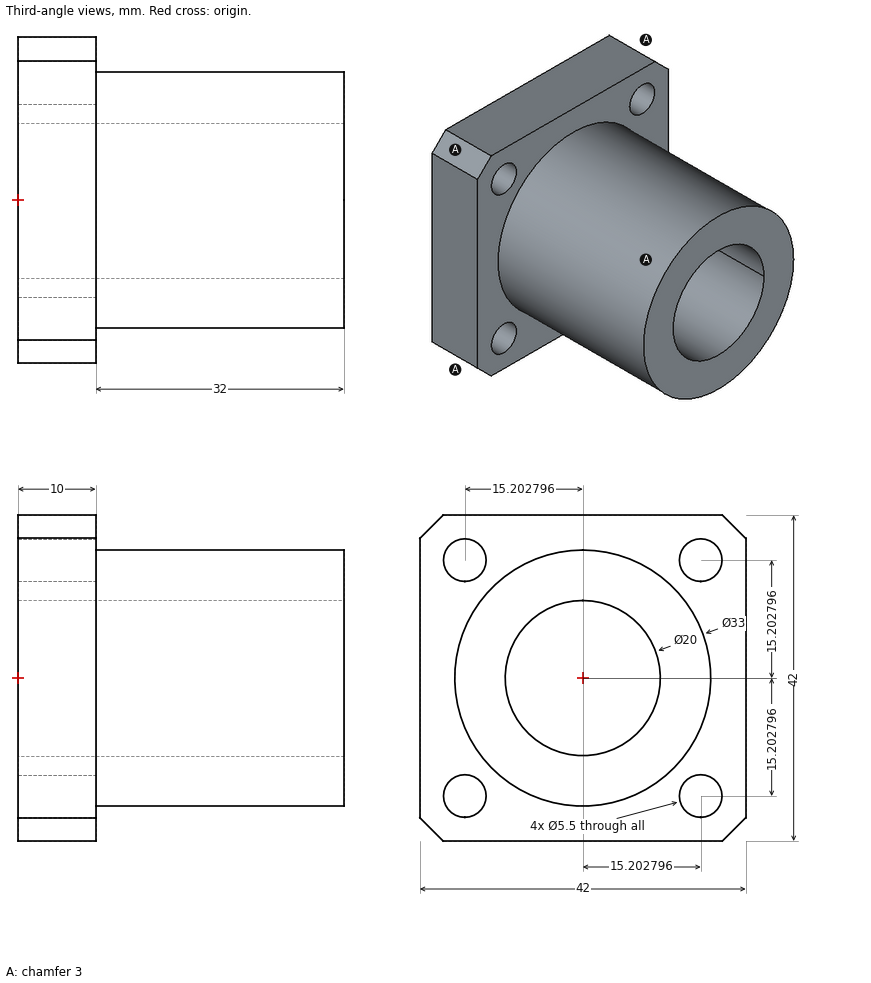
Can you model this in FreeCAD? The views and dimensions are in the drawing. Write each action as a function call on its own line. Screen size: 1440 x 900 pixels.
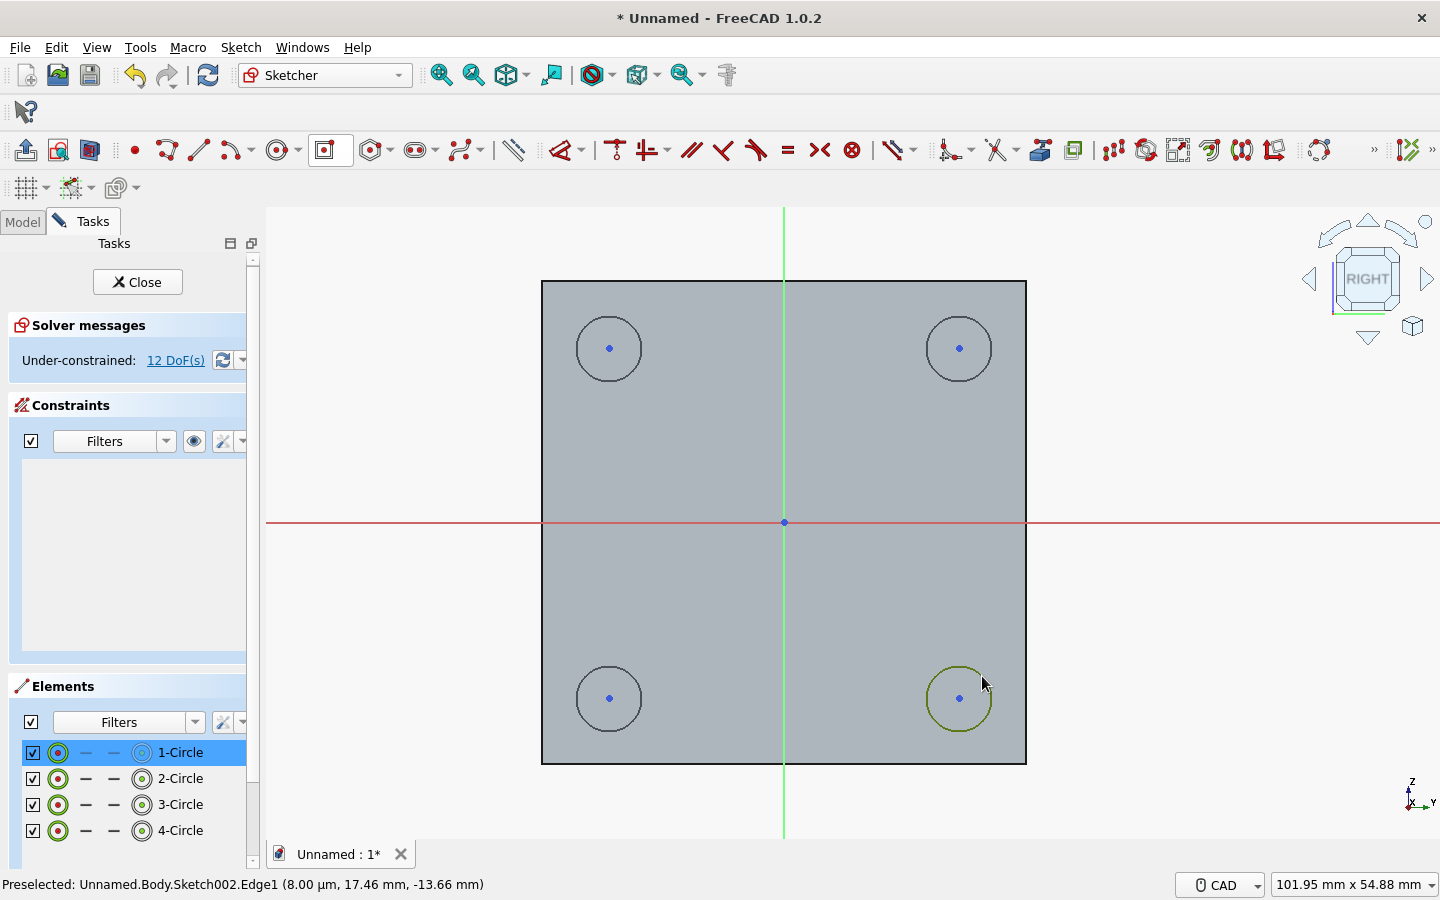
click(982, 326)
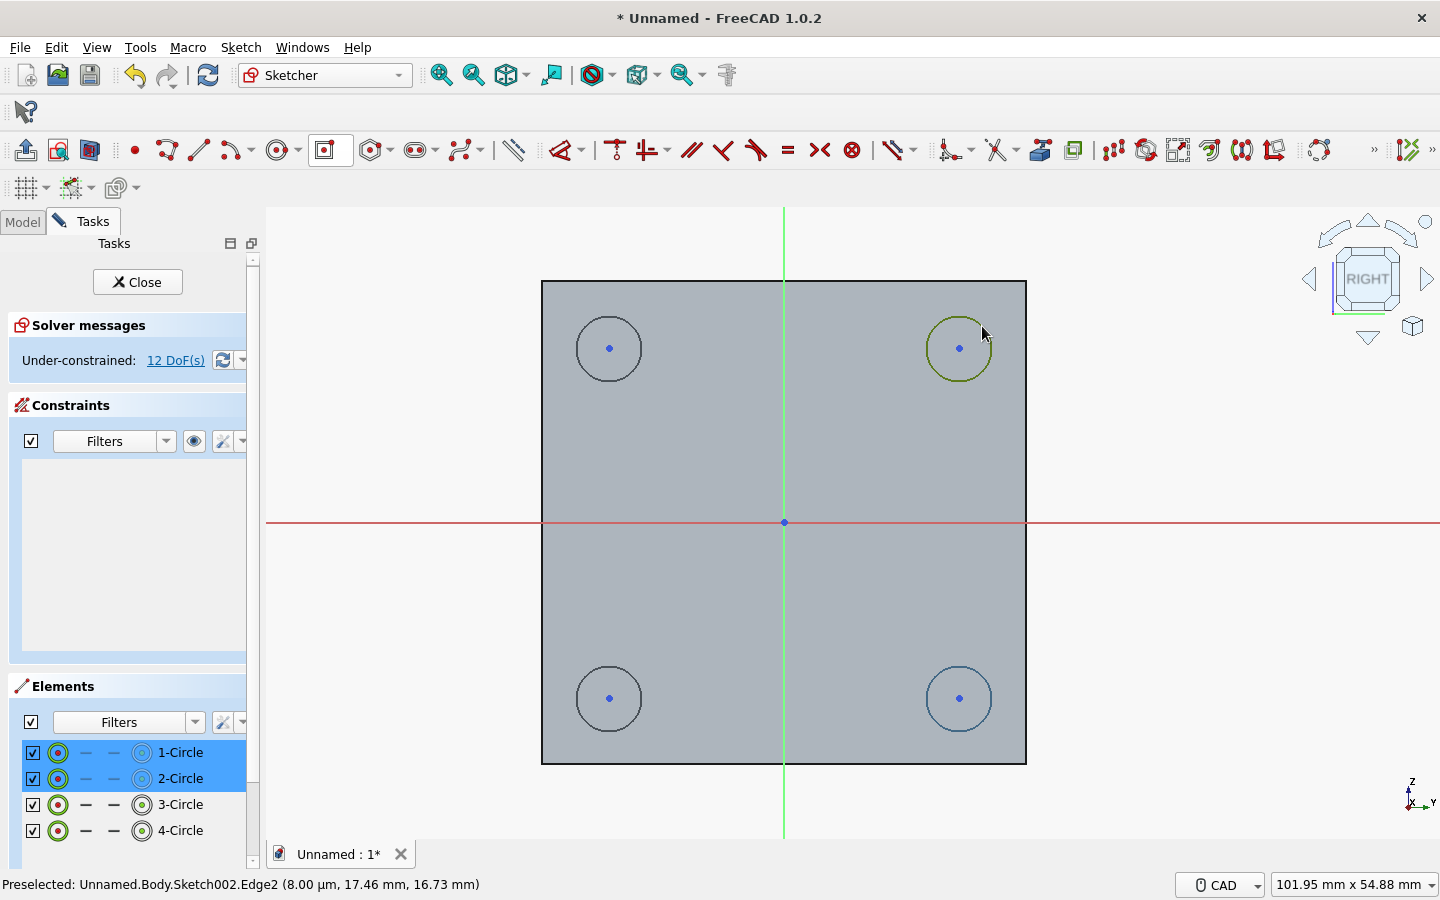
click(632, 326)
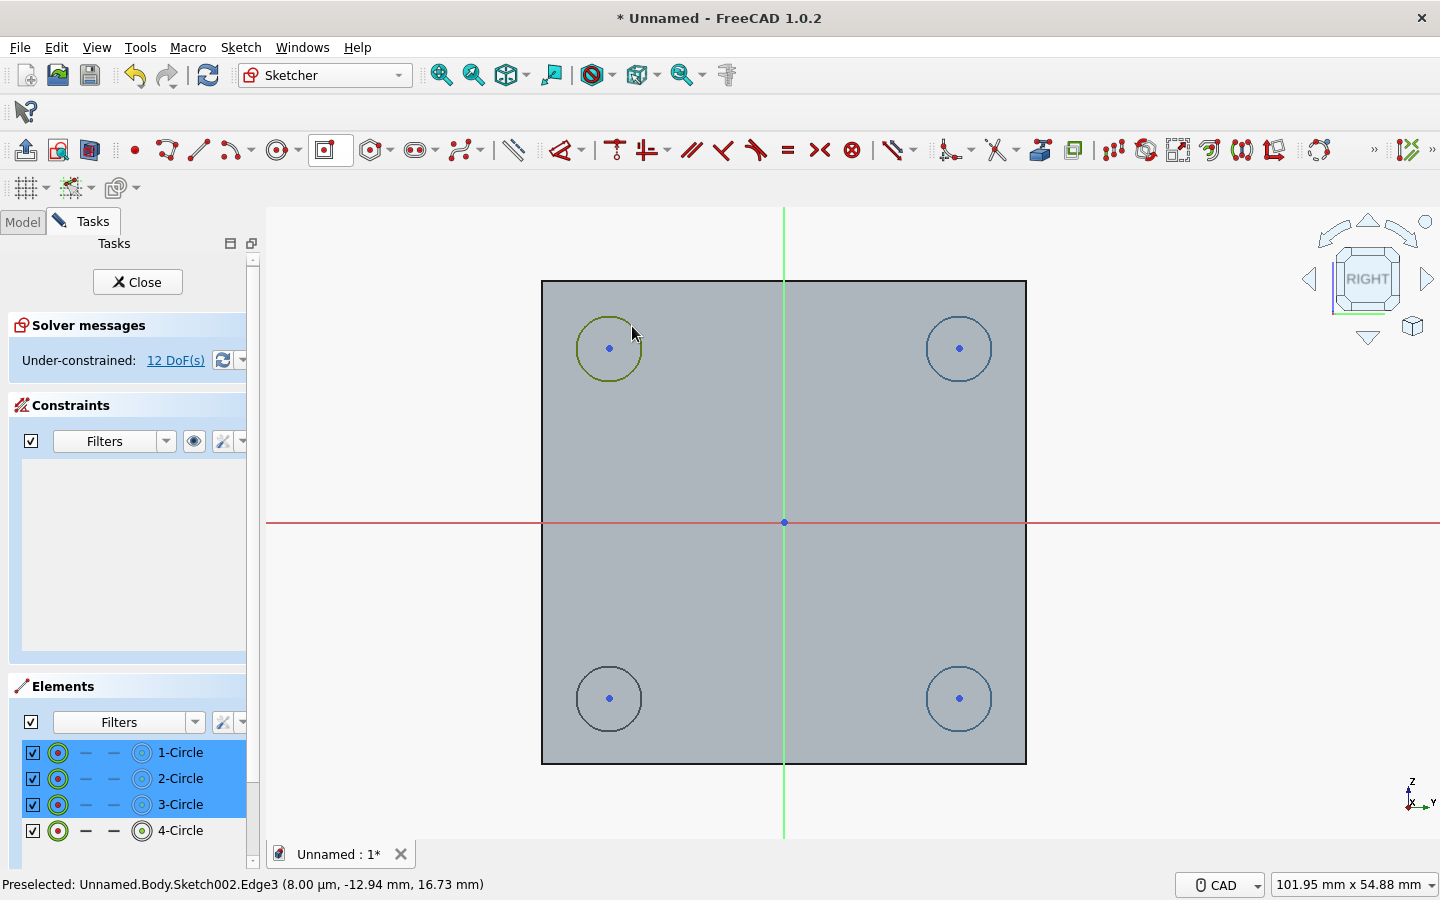
click(632, 676)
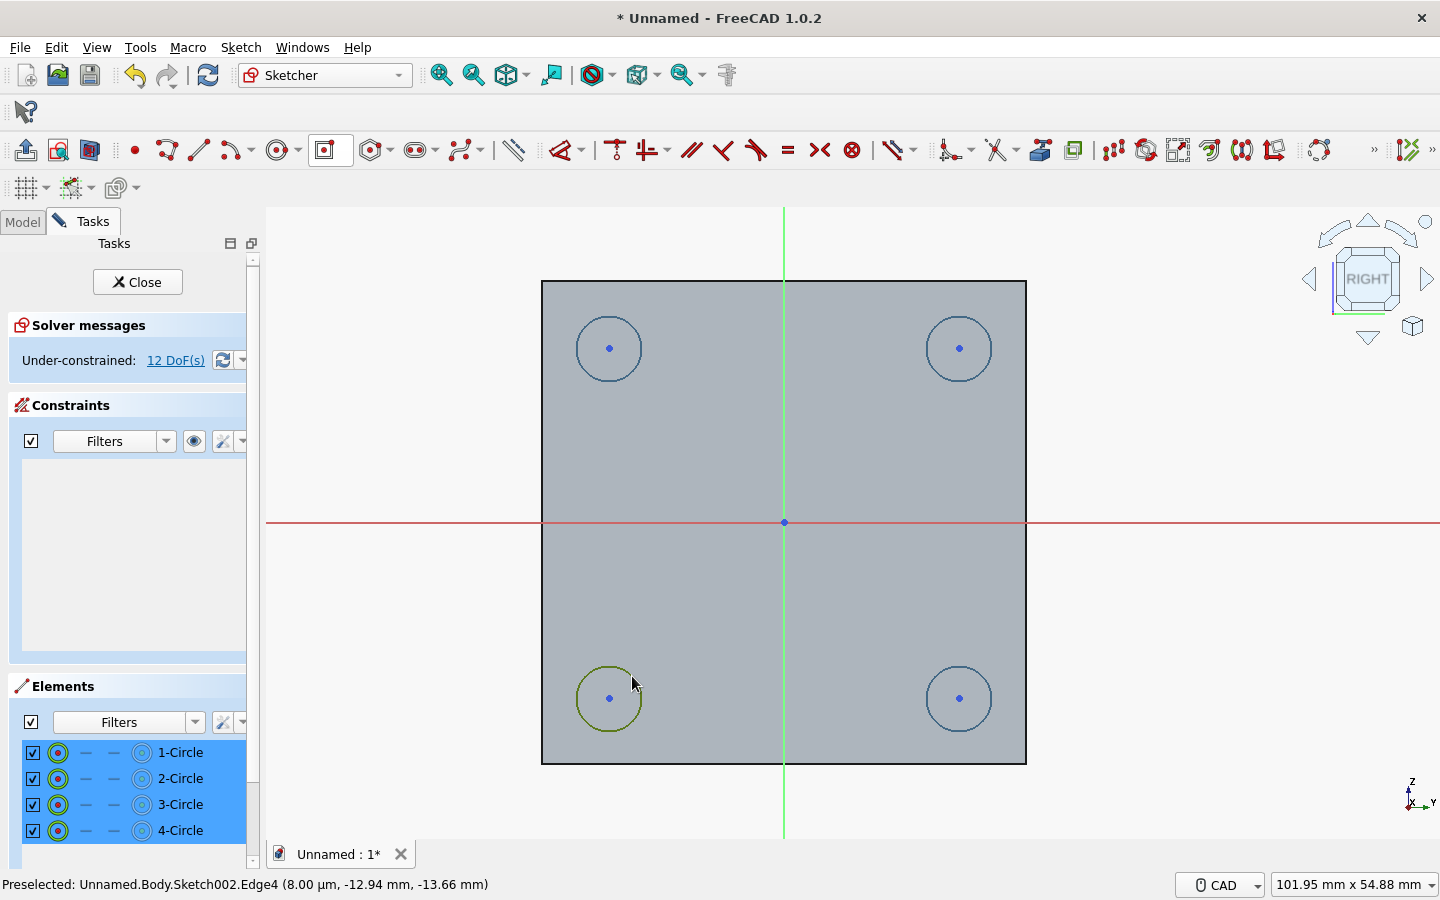
click(788, 150)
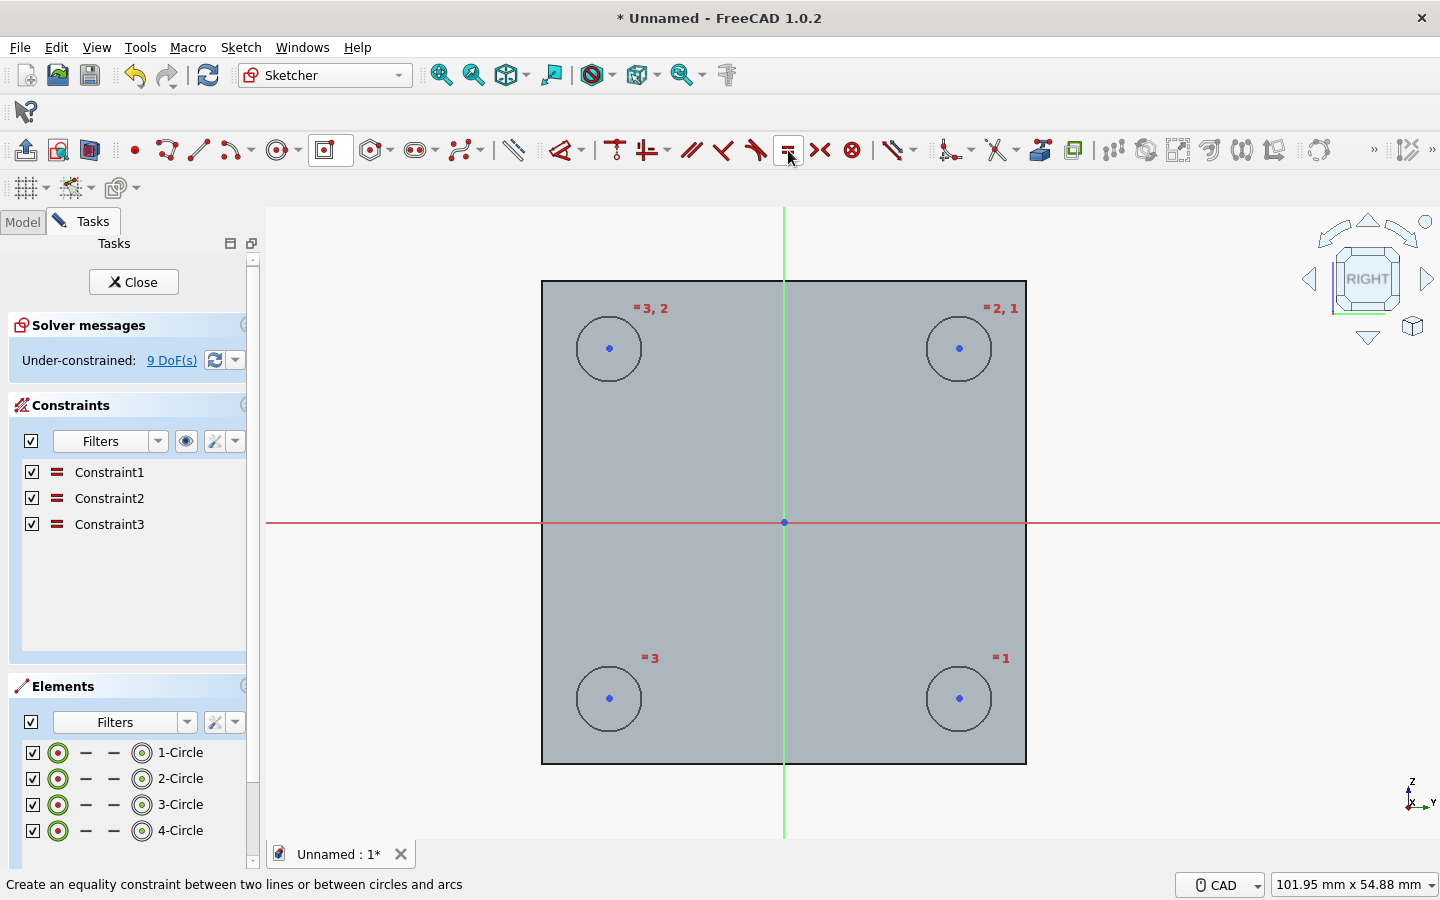
click(560, 150)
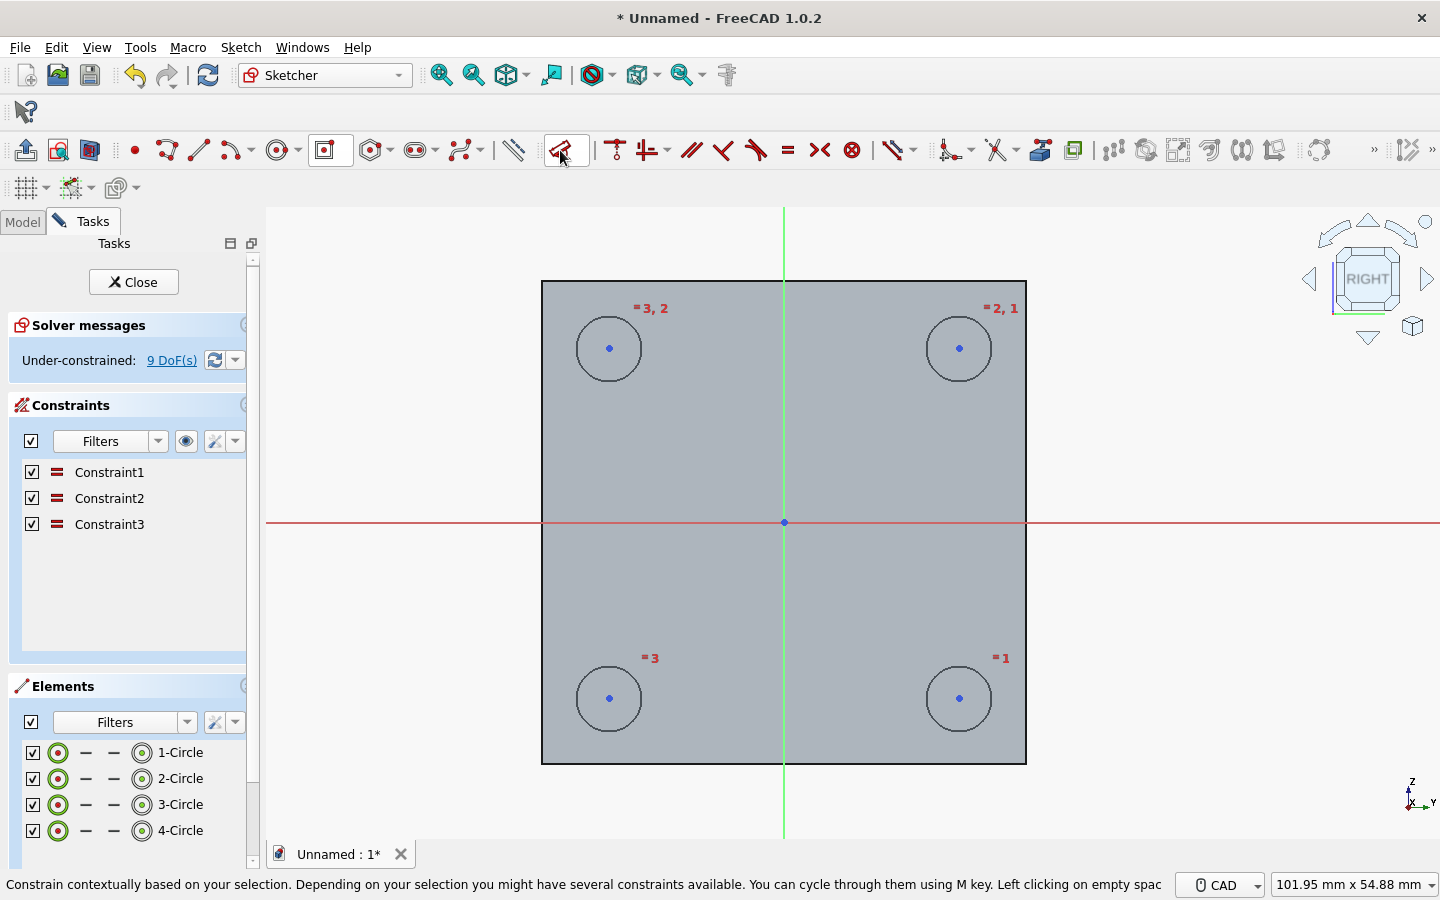
click(982, 676)
click(1005, 653)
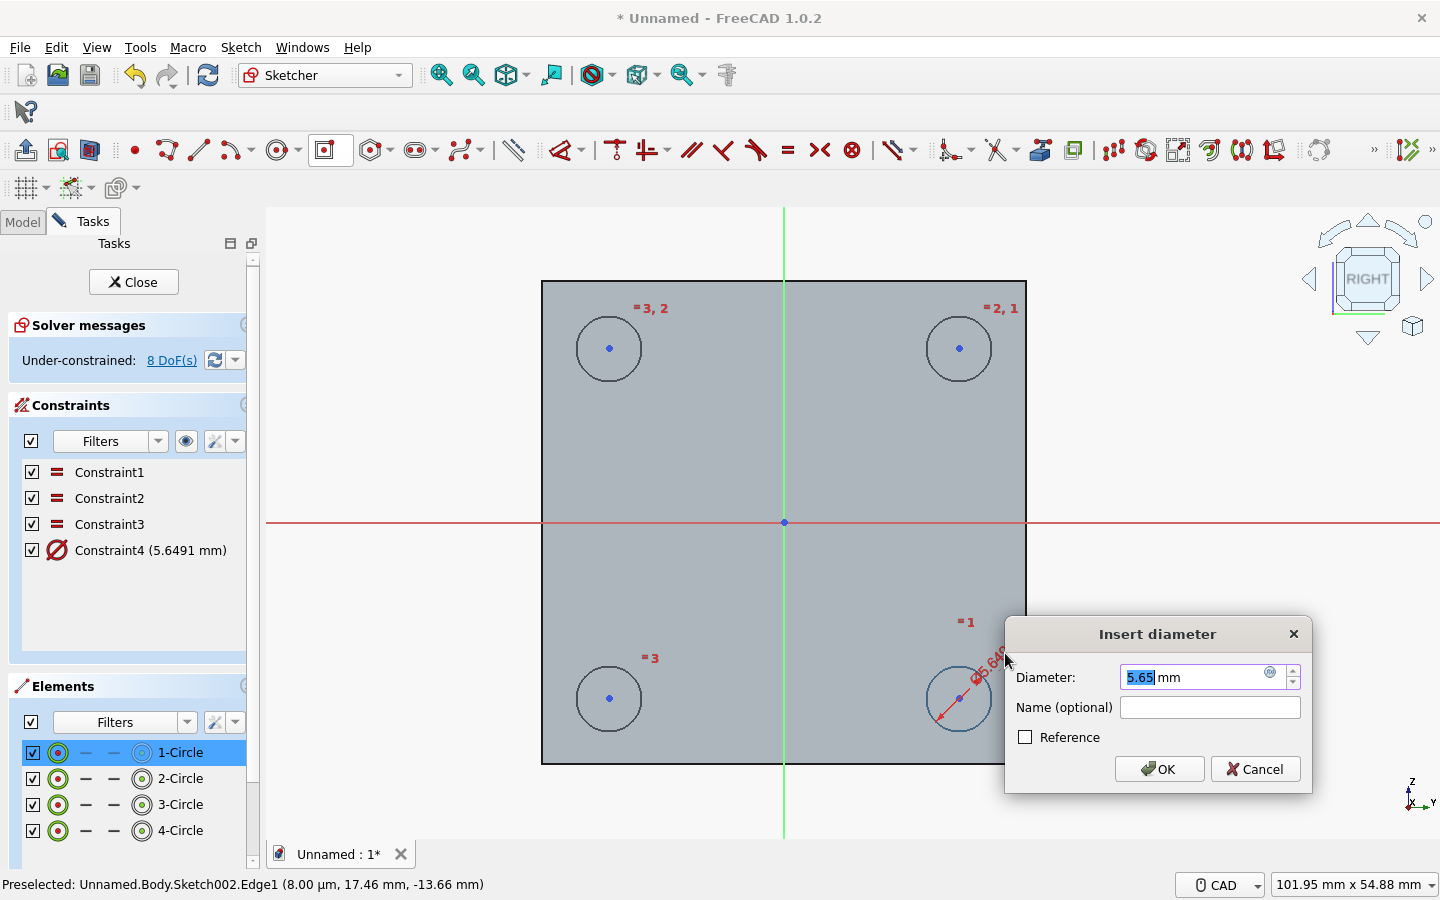
text(5.5)
key(Return)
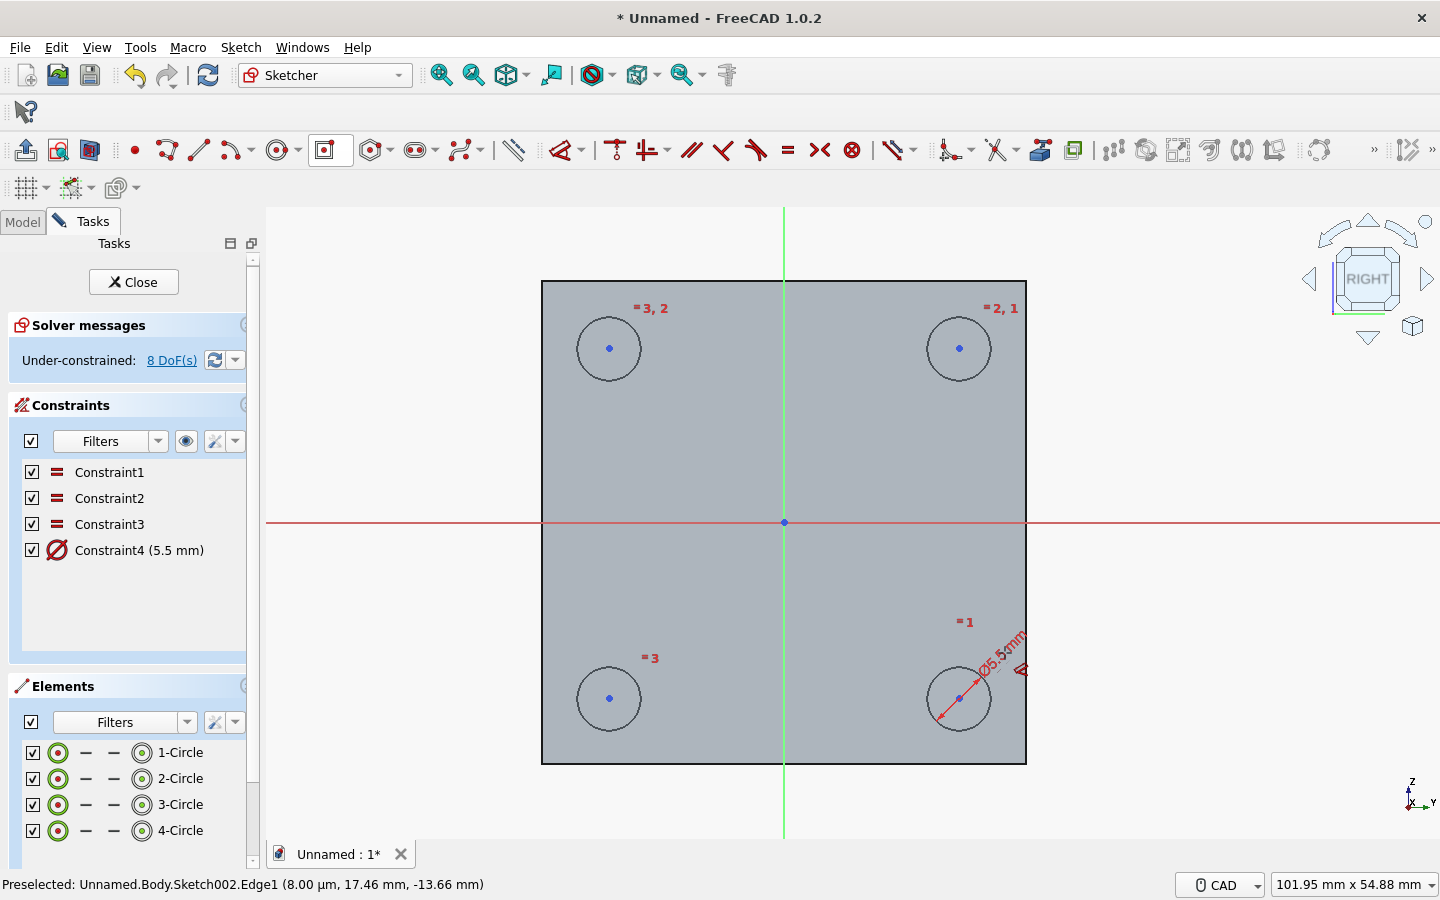
click(959, 699)
click(872, 733)